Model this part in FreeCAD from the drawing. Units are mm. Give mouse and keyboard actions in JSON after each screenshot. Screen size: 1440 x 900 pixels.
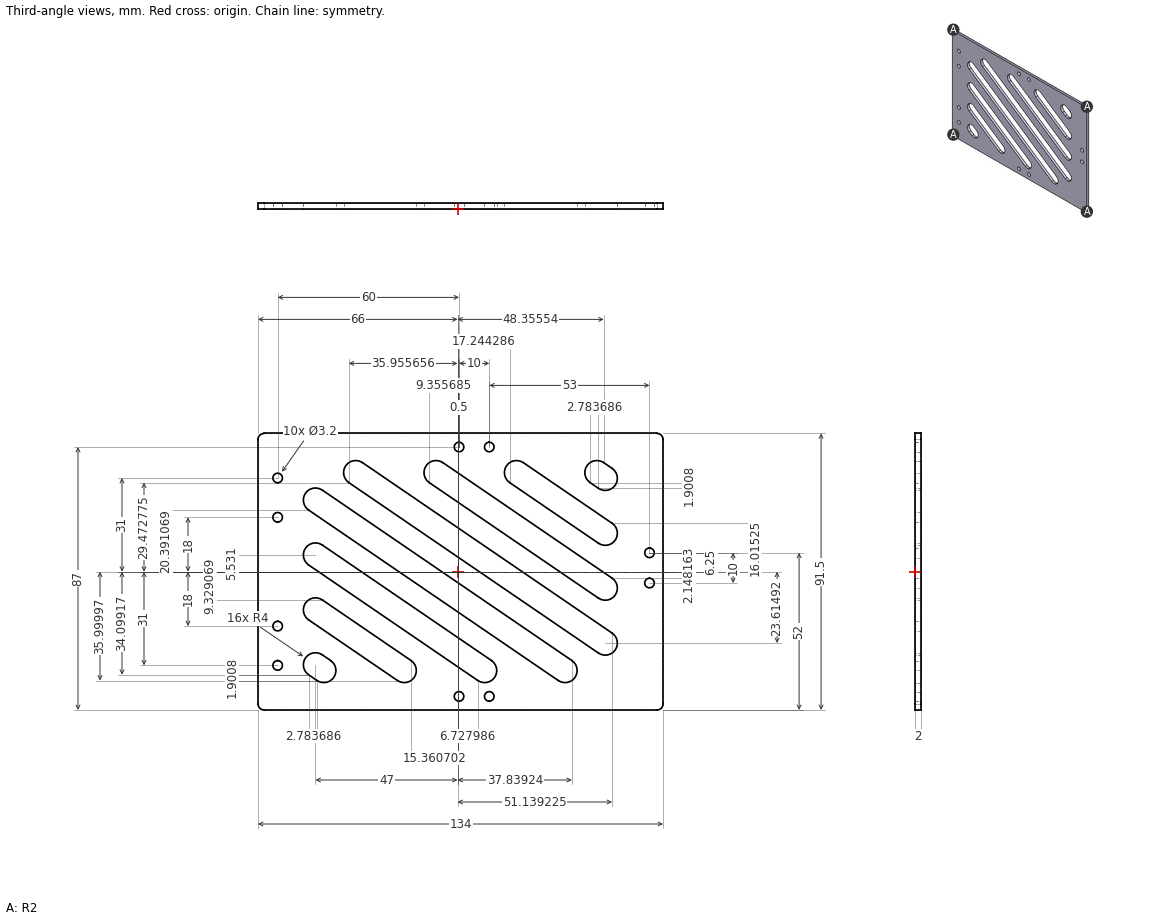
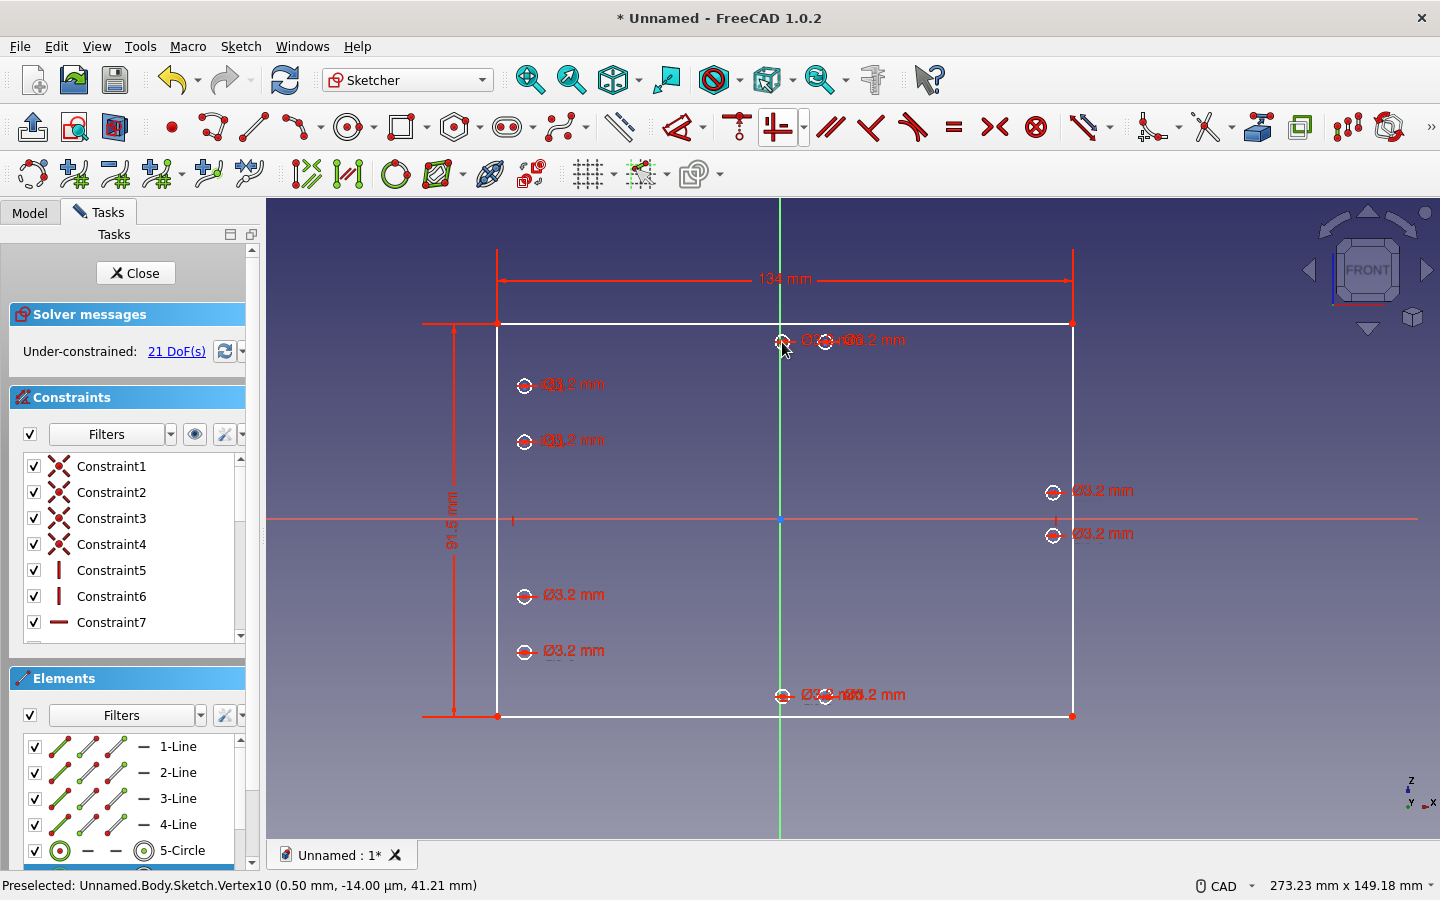
{"action": "left_click", "coordinate": [825, 342]}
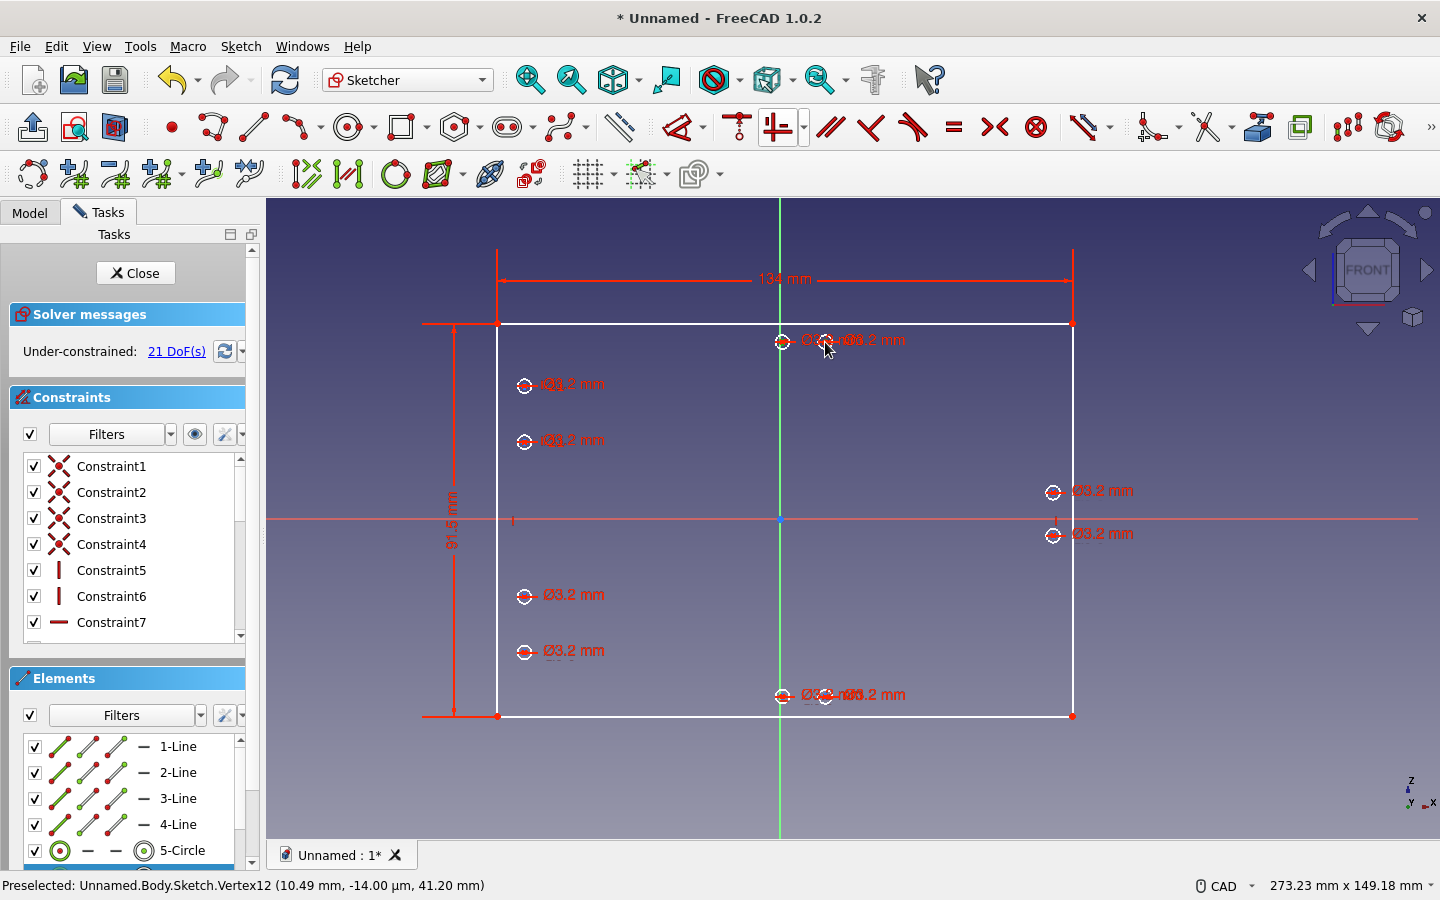
{"action": "left_click", "coordinate": [804, 128]}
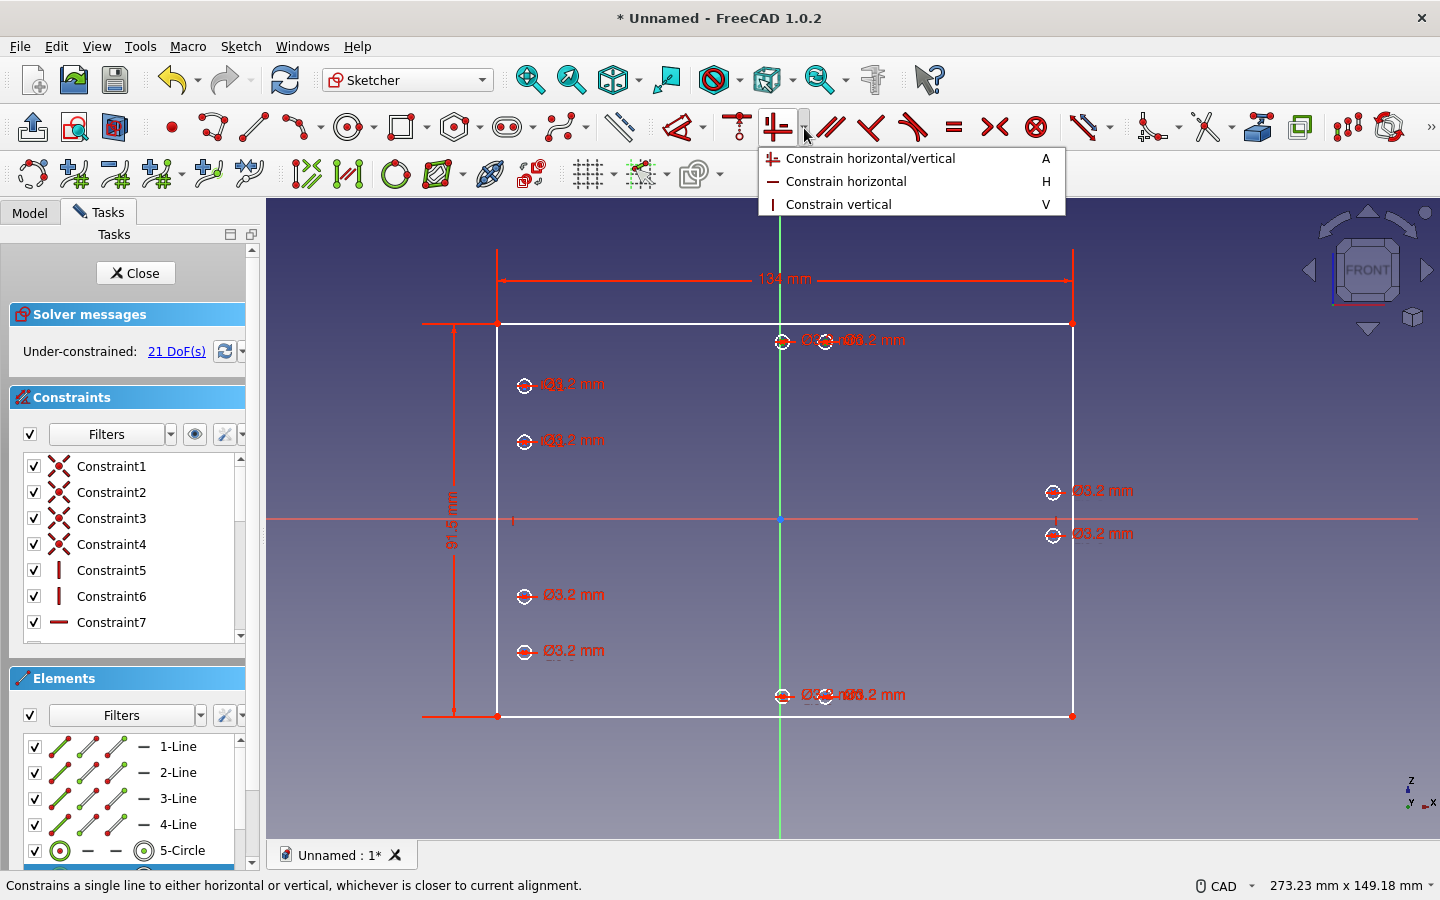
{"action": "left_click", "coordinate": [912, 182]}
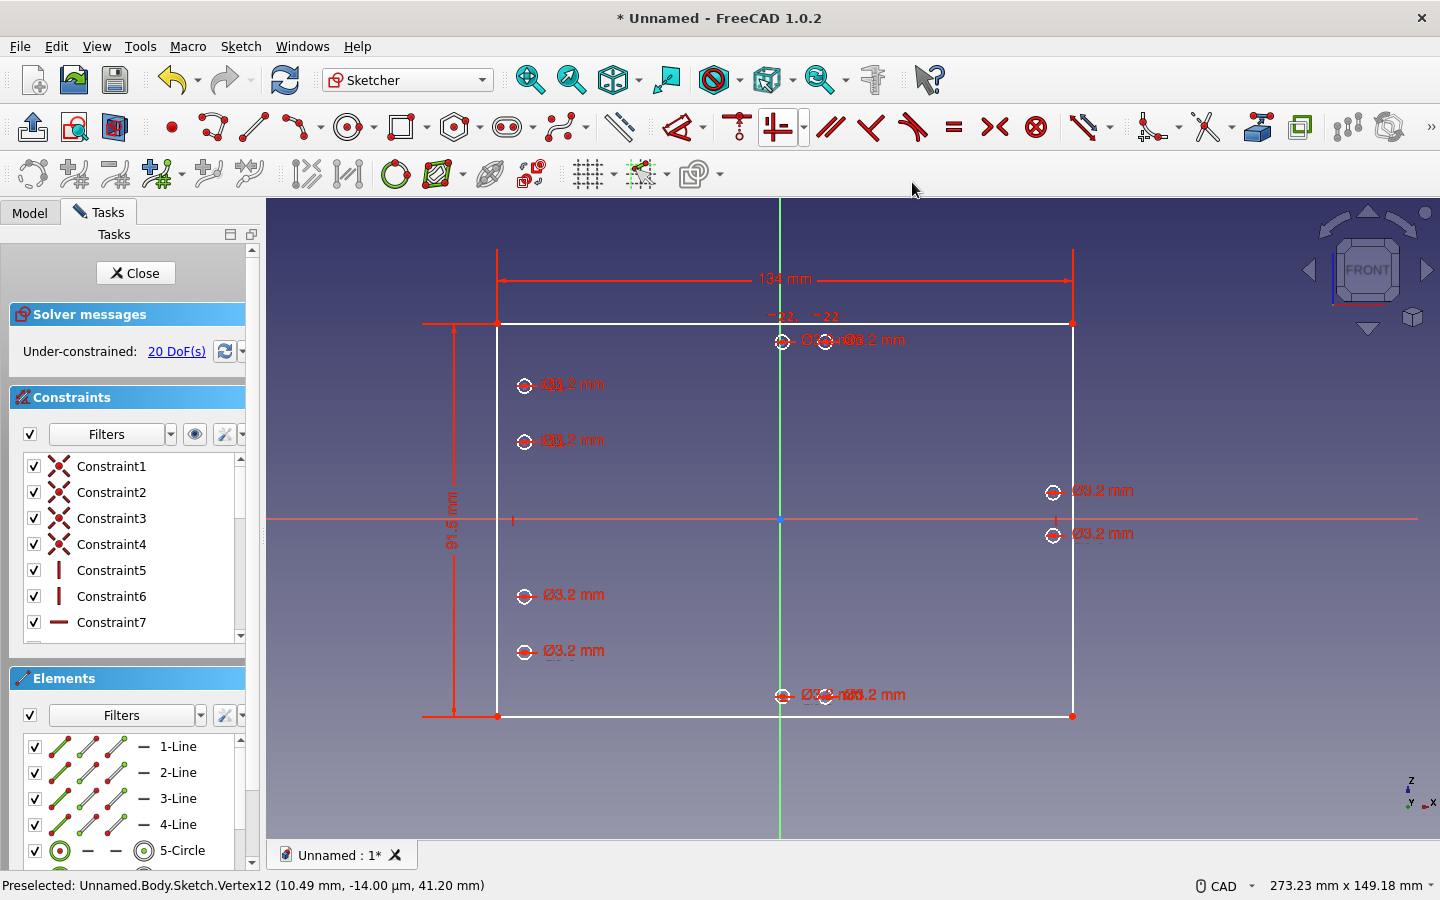
{"action": "left_click", "coordinate": [525, 442]}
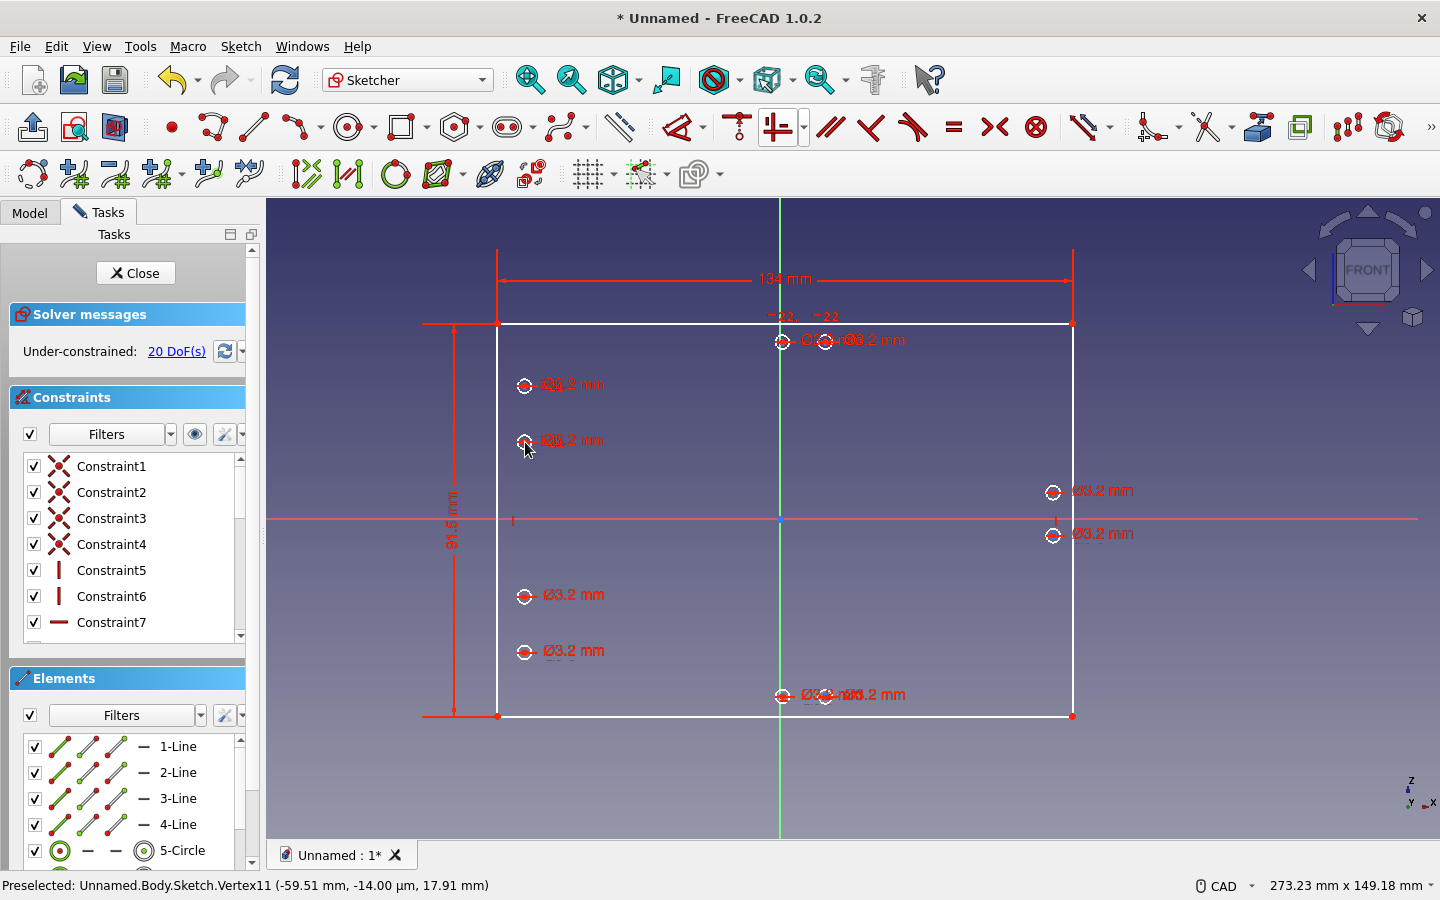
{"action": "left_click", "coordinate": [524, 597]}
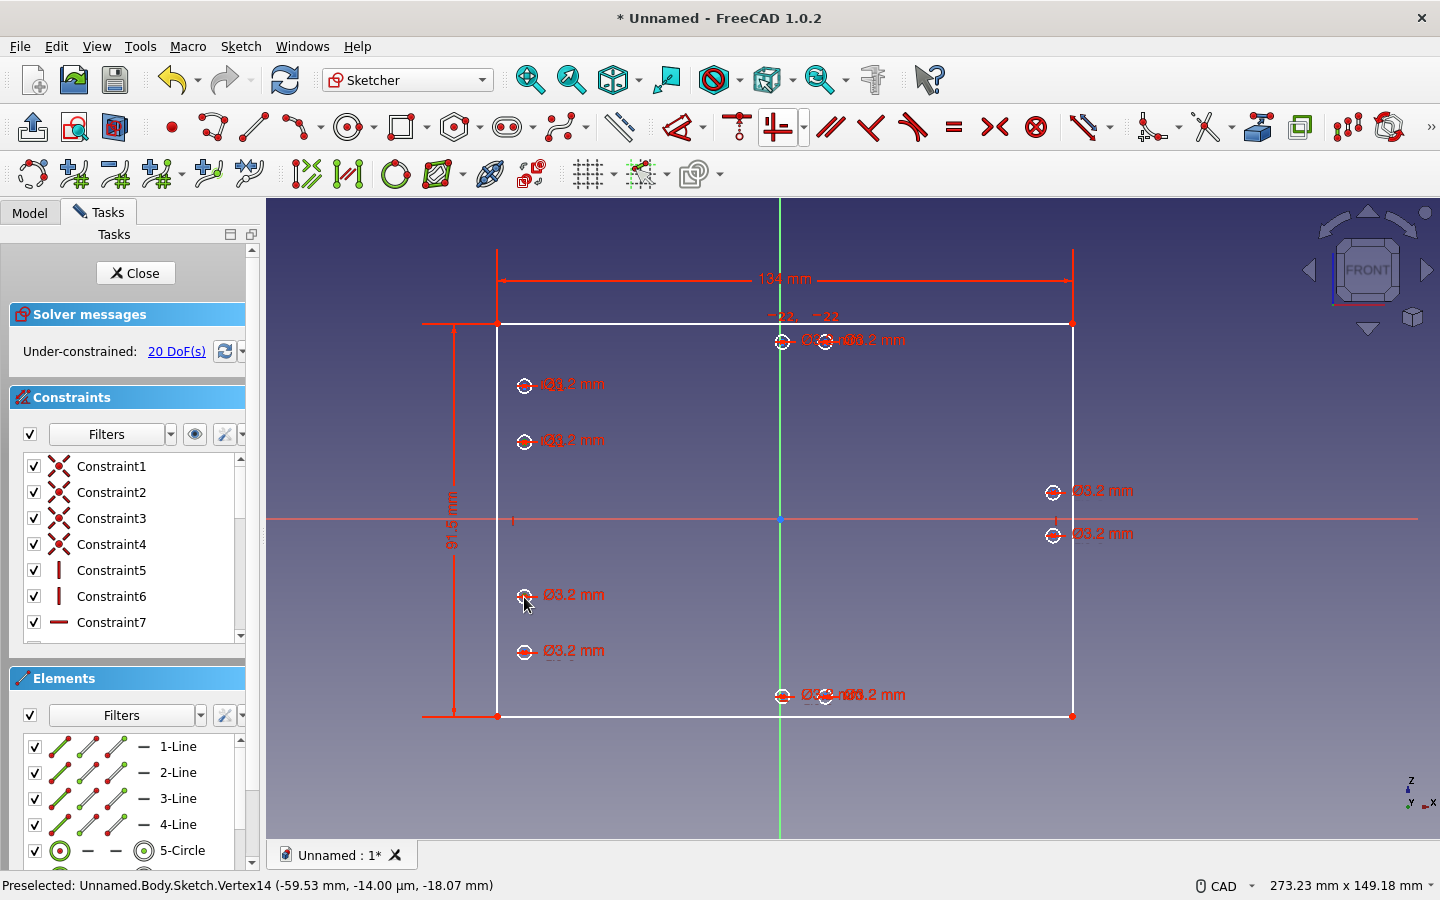
{"action": "left_click", "coordinate": [804, 128]}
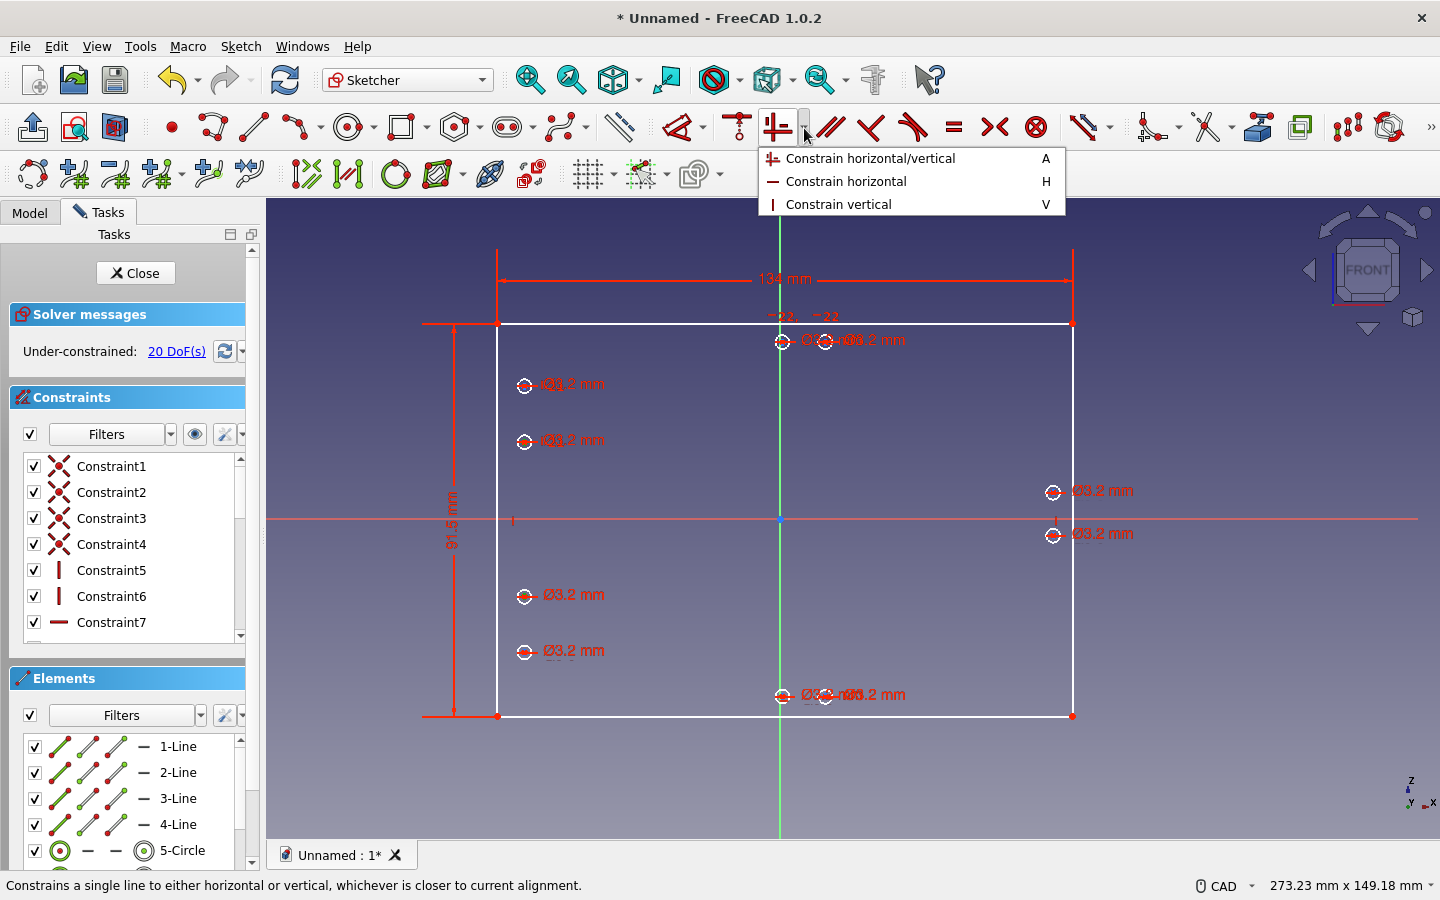
{"action": "left_click", "coordinate": [912, 204]}